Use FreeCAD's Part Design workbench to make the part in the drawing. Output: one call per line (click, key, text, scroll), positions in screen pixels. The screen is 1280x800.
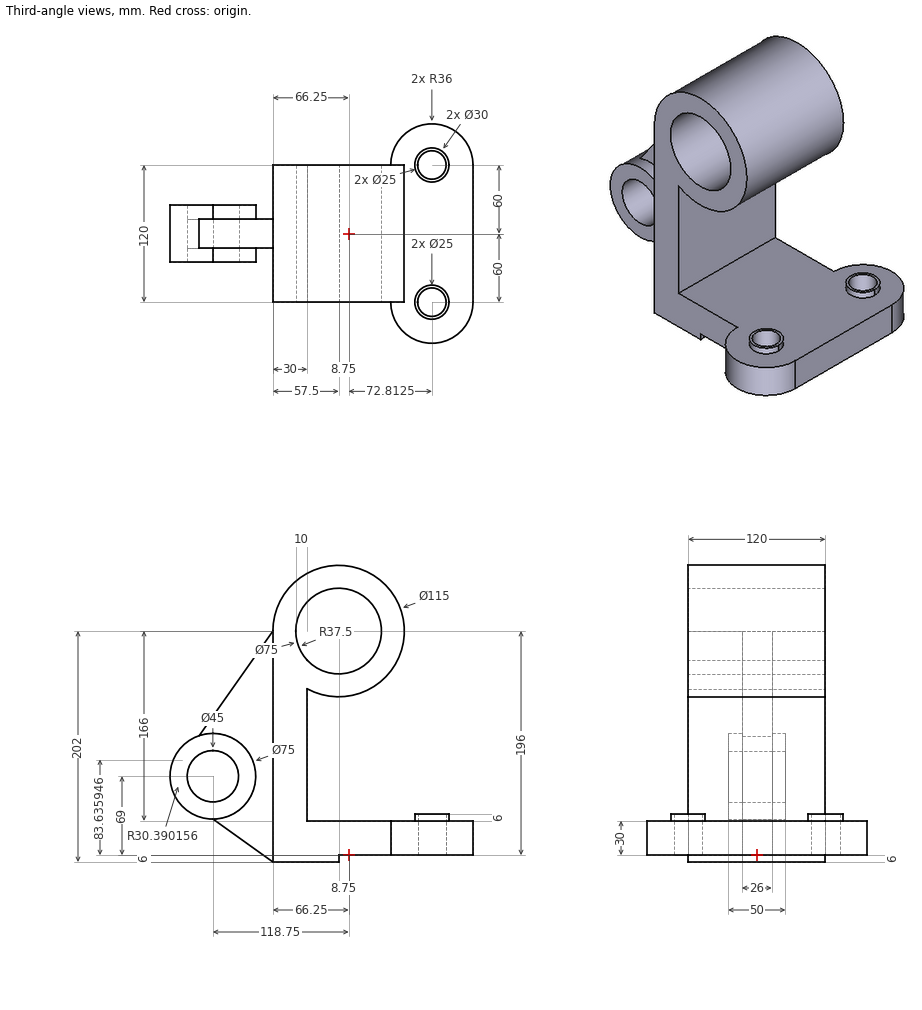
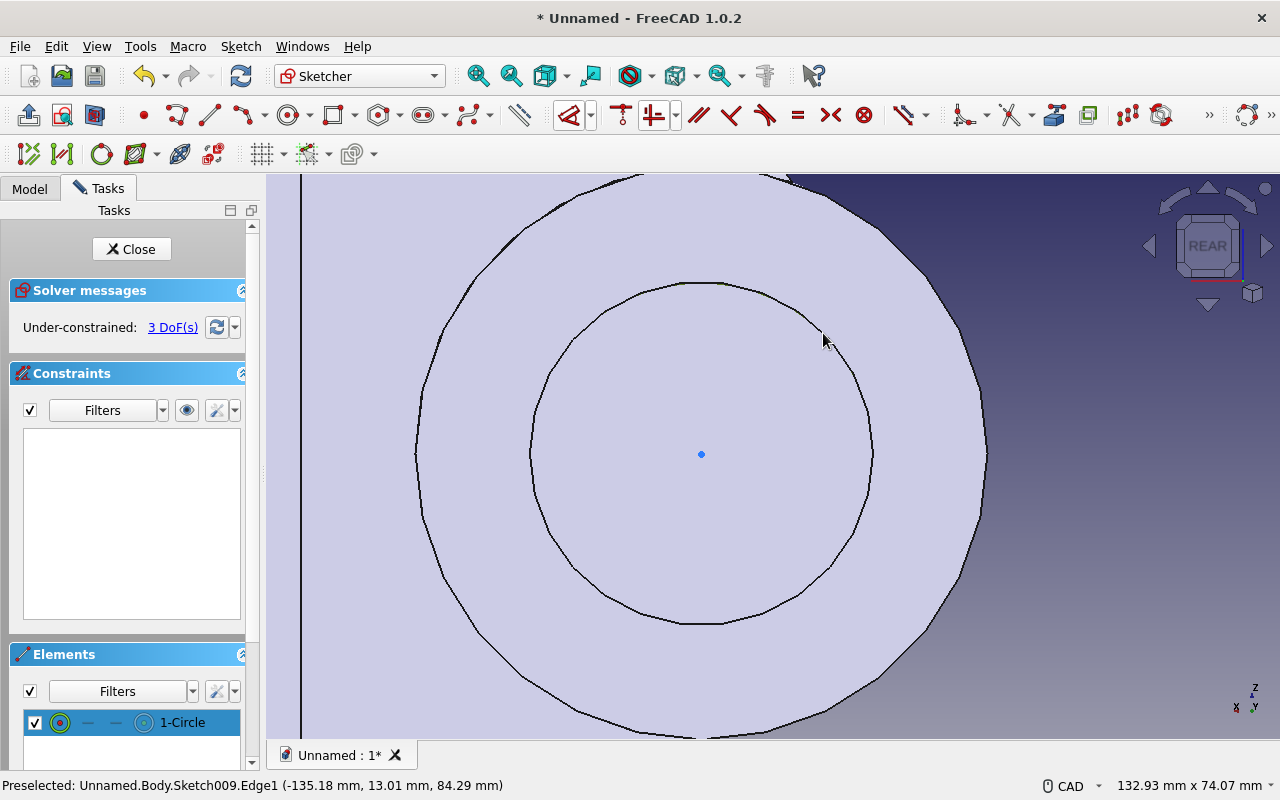
key(k)
key(o)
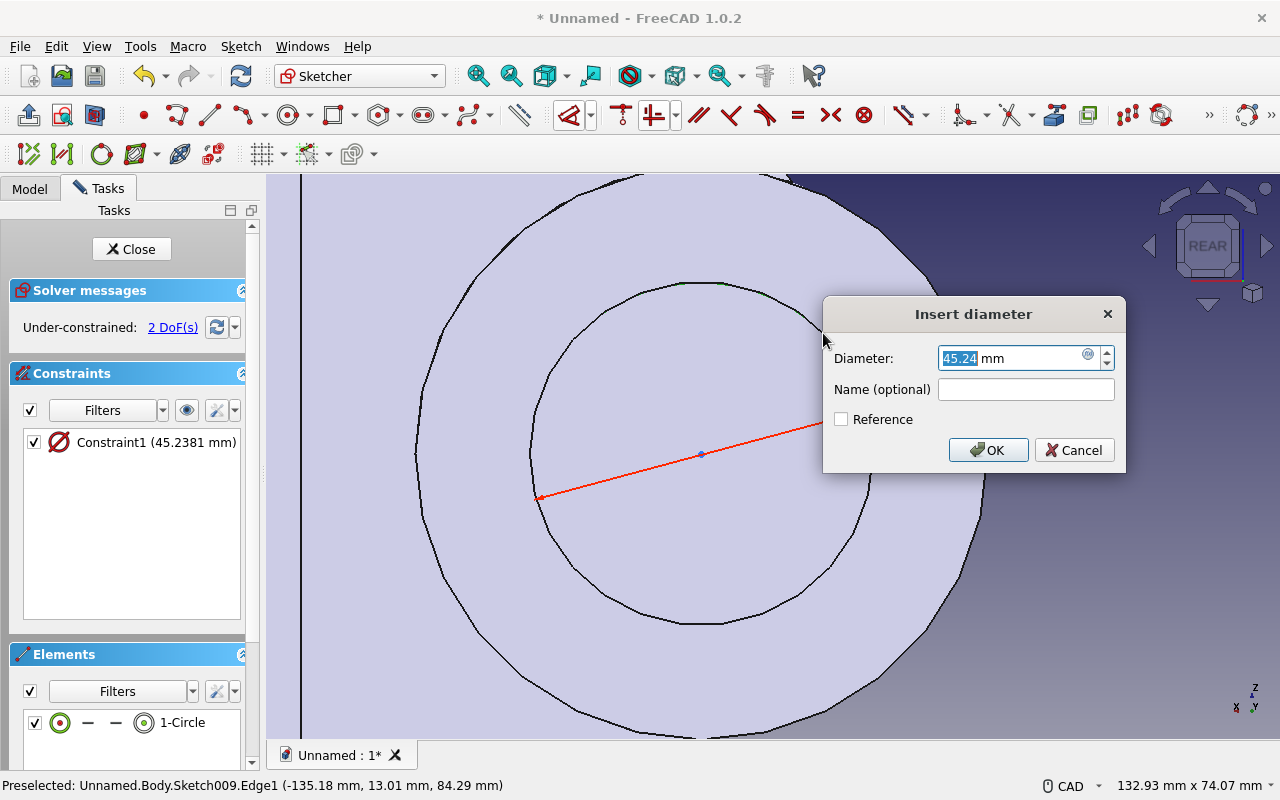
text(45)
key(Return)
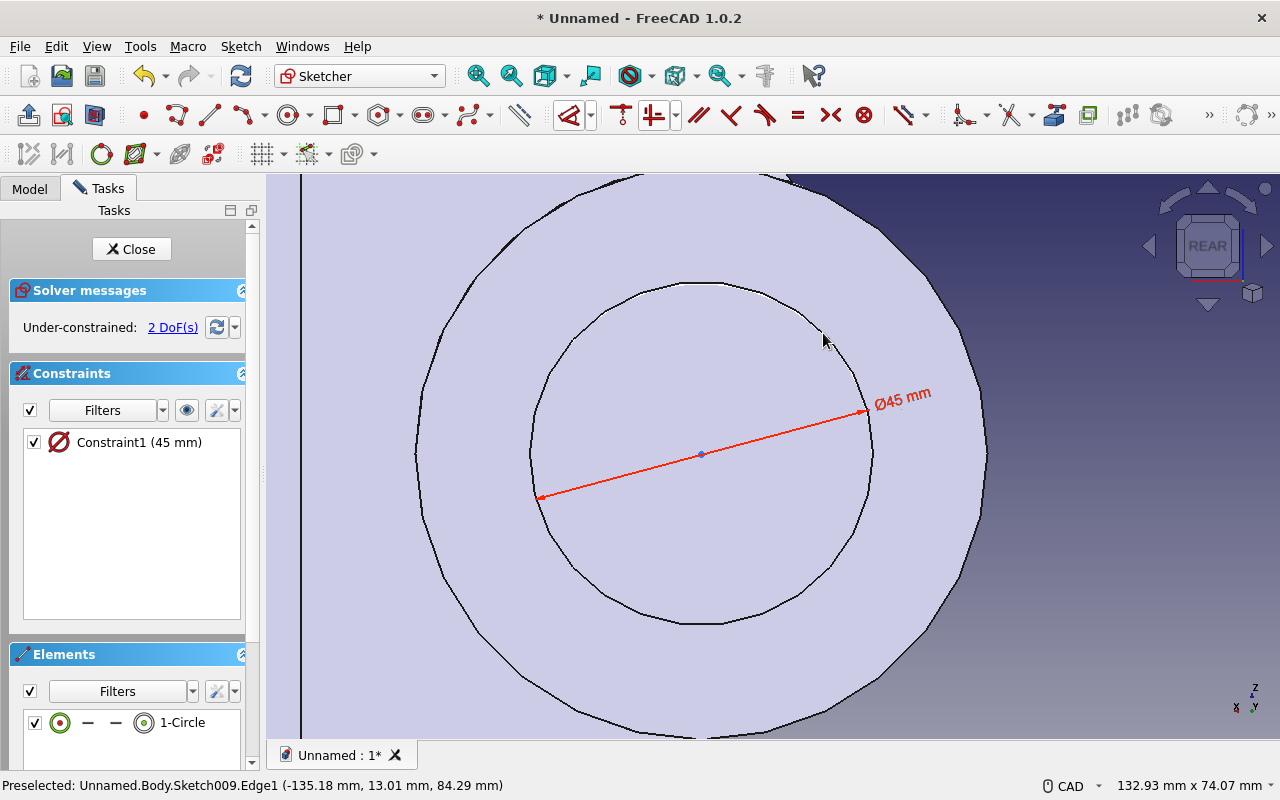
click(701, 455)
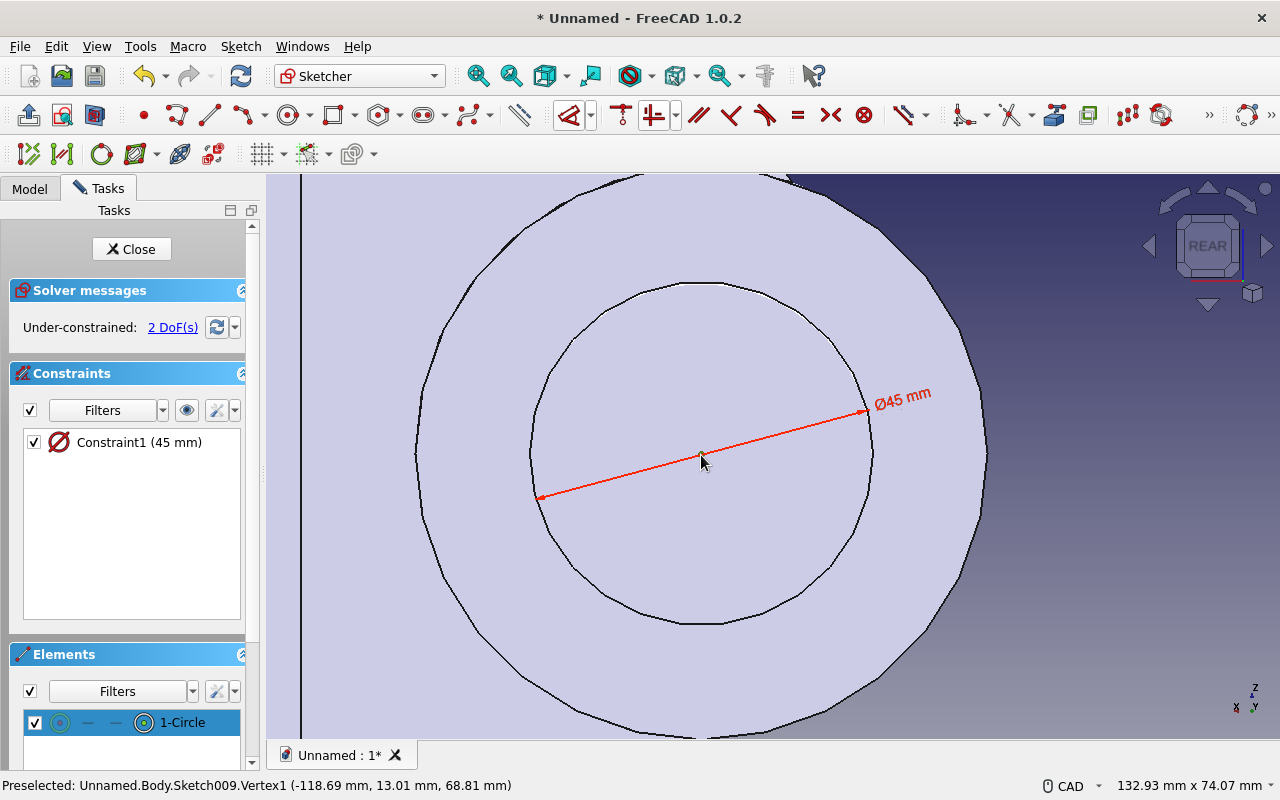
key(i)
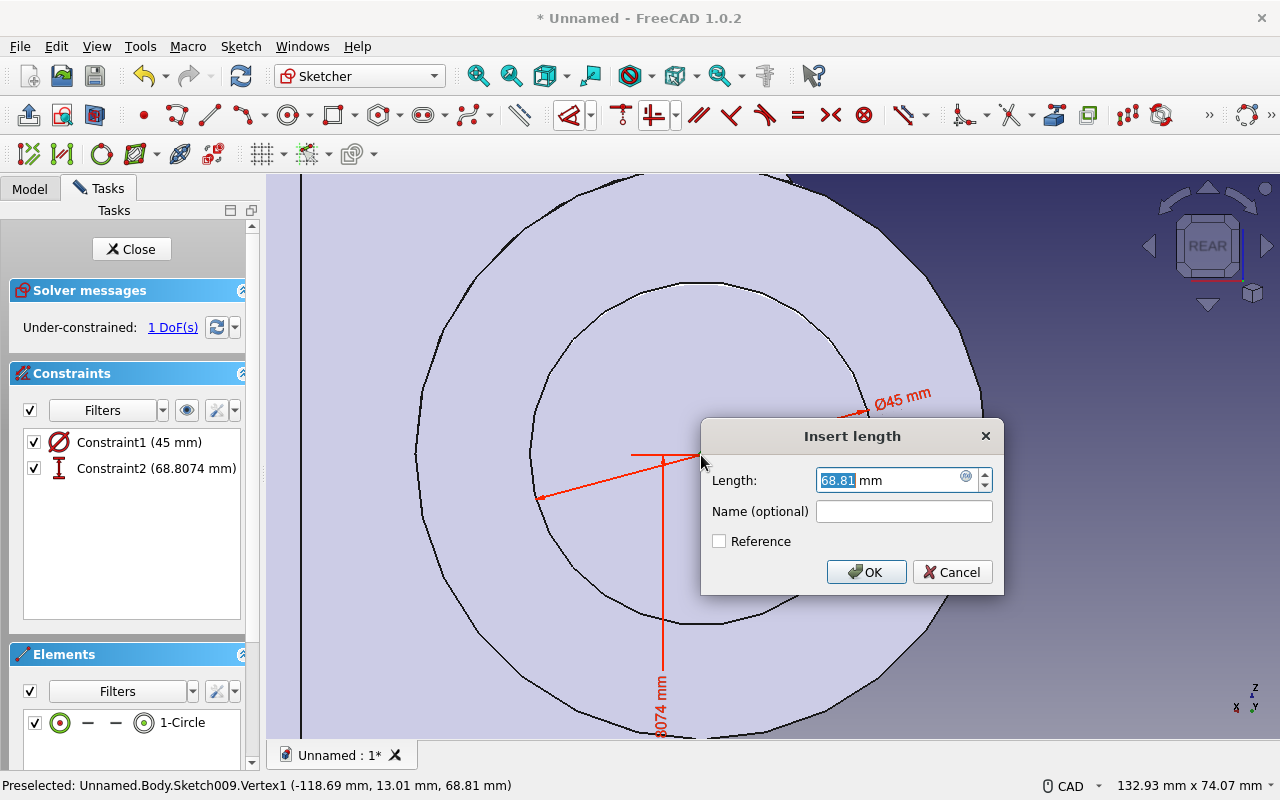
text(69)
key(Return)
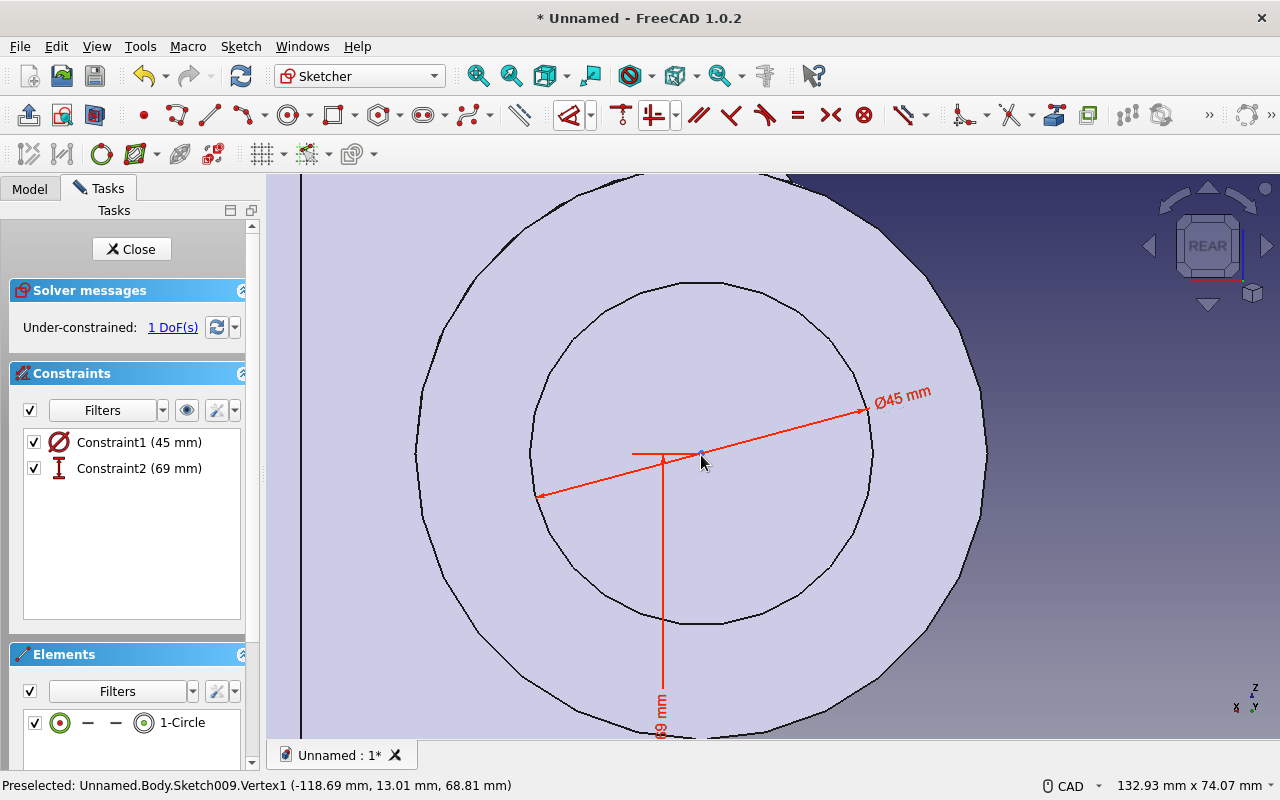
click(701, 454)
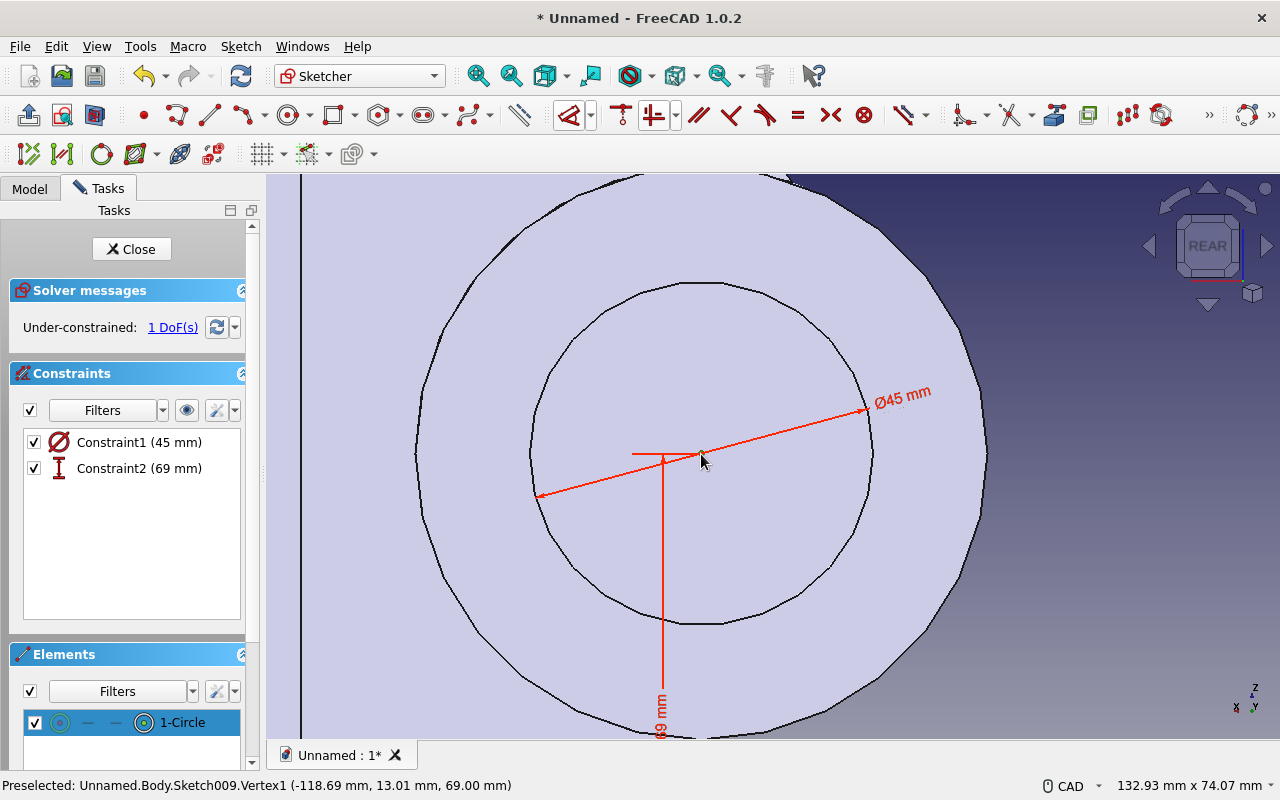
click(590, 116)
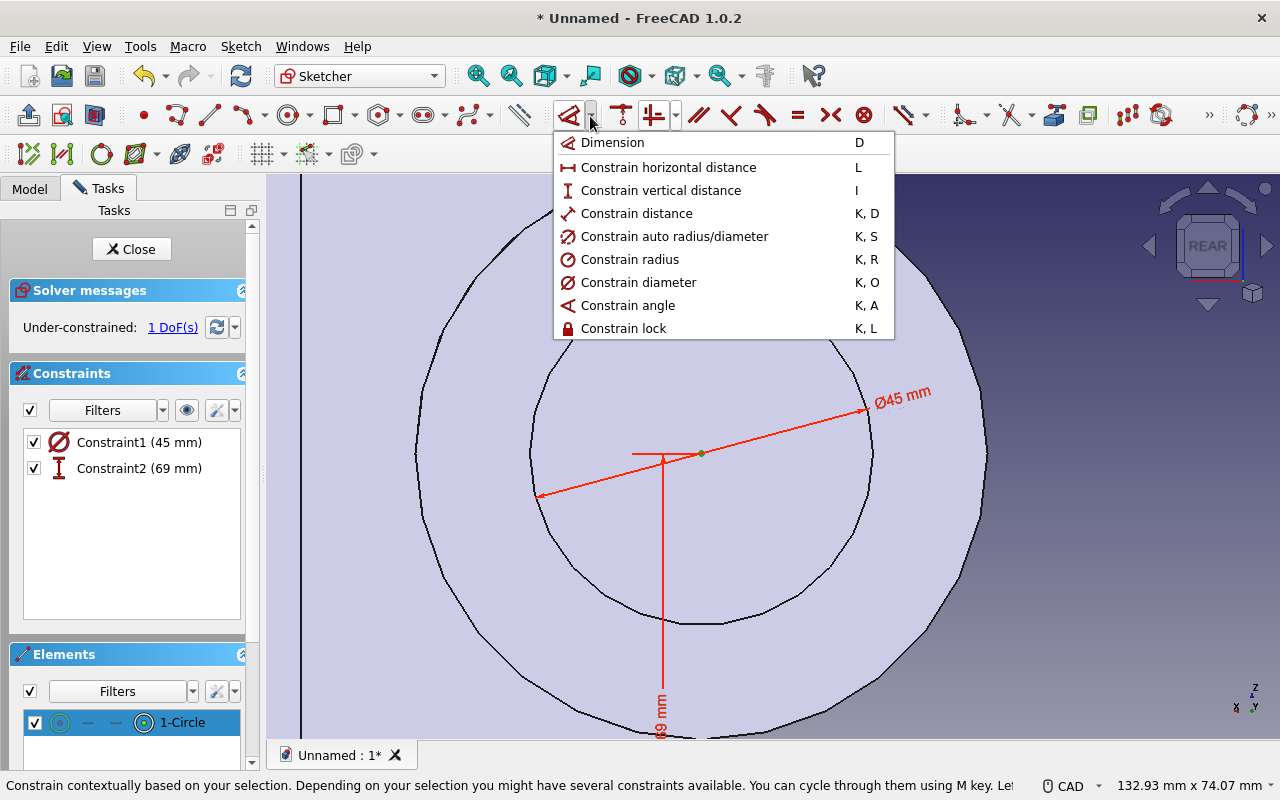
click(724, 168)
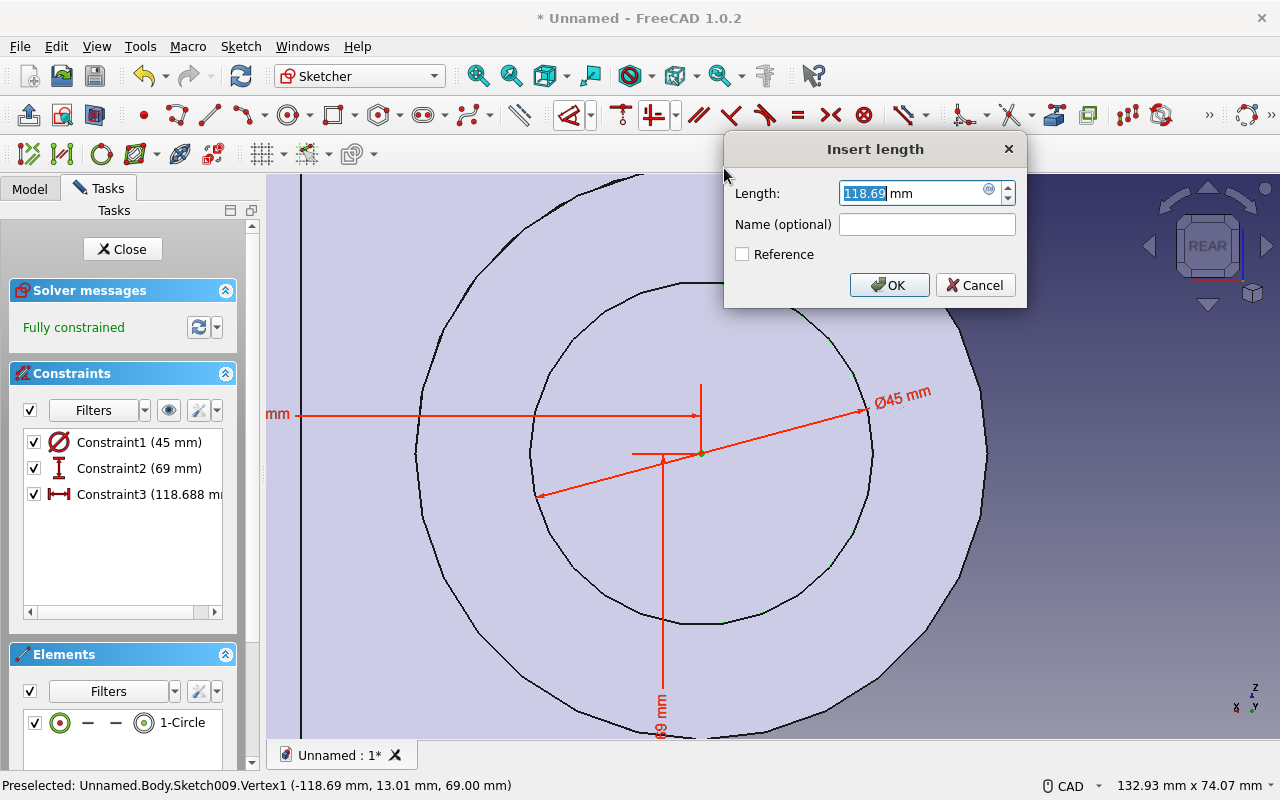
text(118.75)
key(Return)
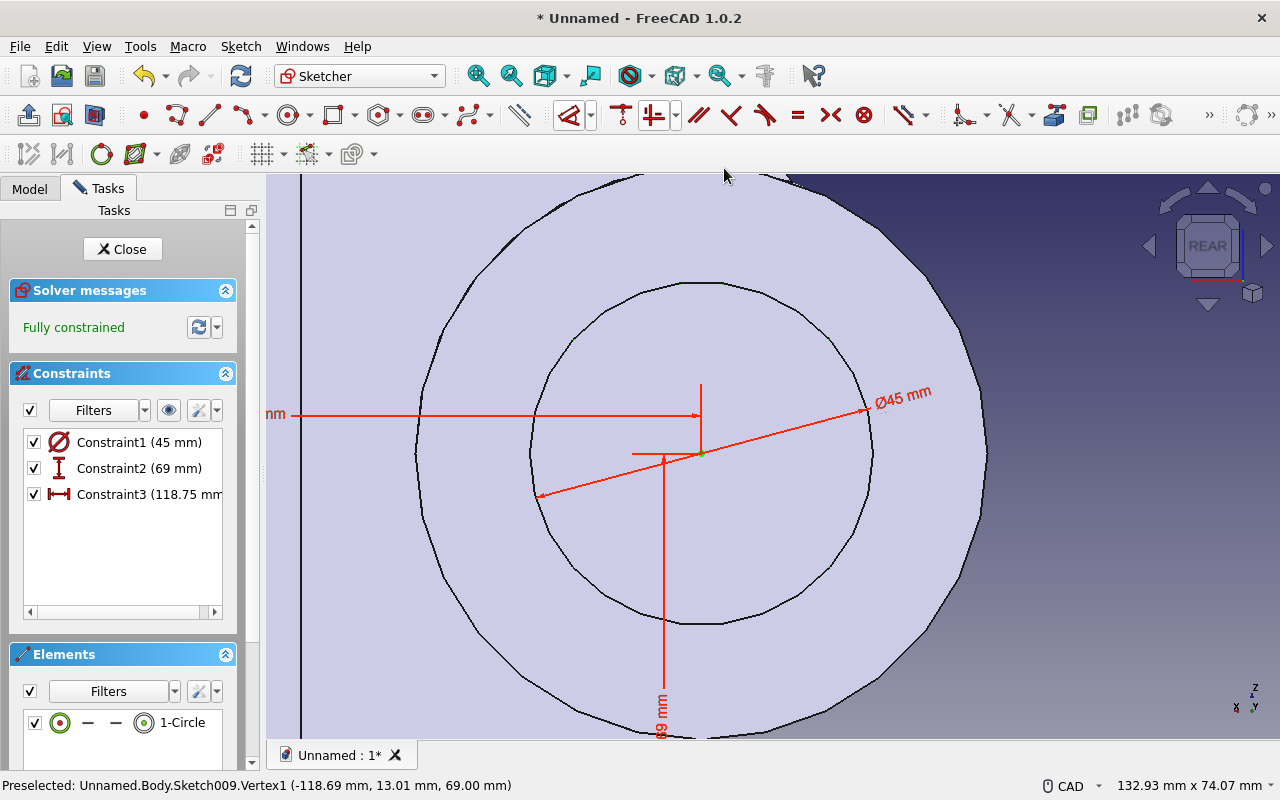
click(123, 249)